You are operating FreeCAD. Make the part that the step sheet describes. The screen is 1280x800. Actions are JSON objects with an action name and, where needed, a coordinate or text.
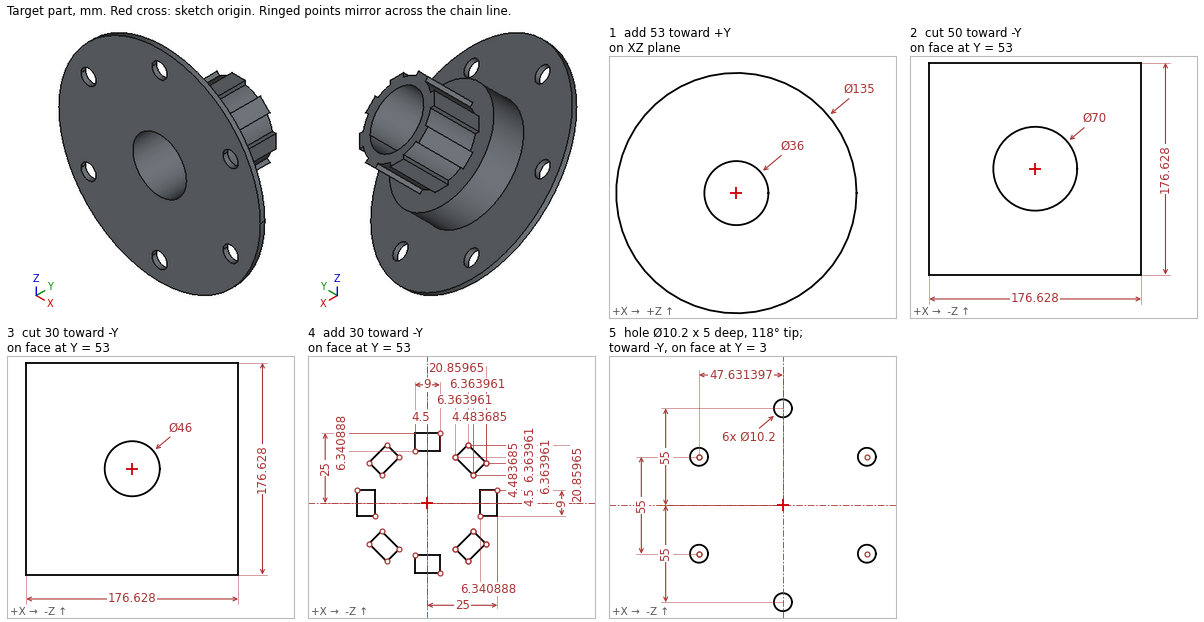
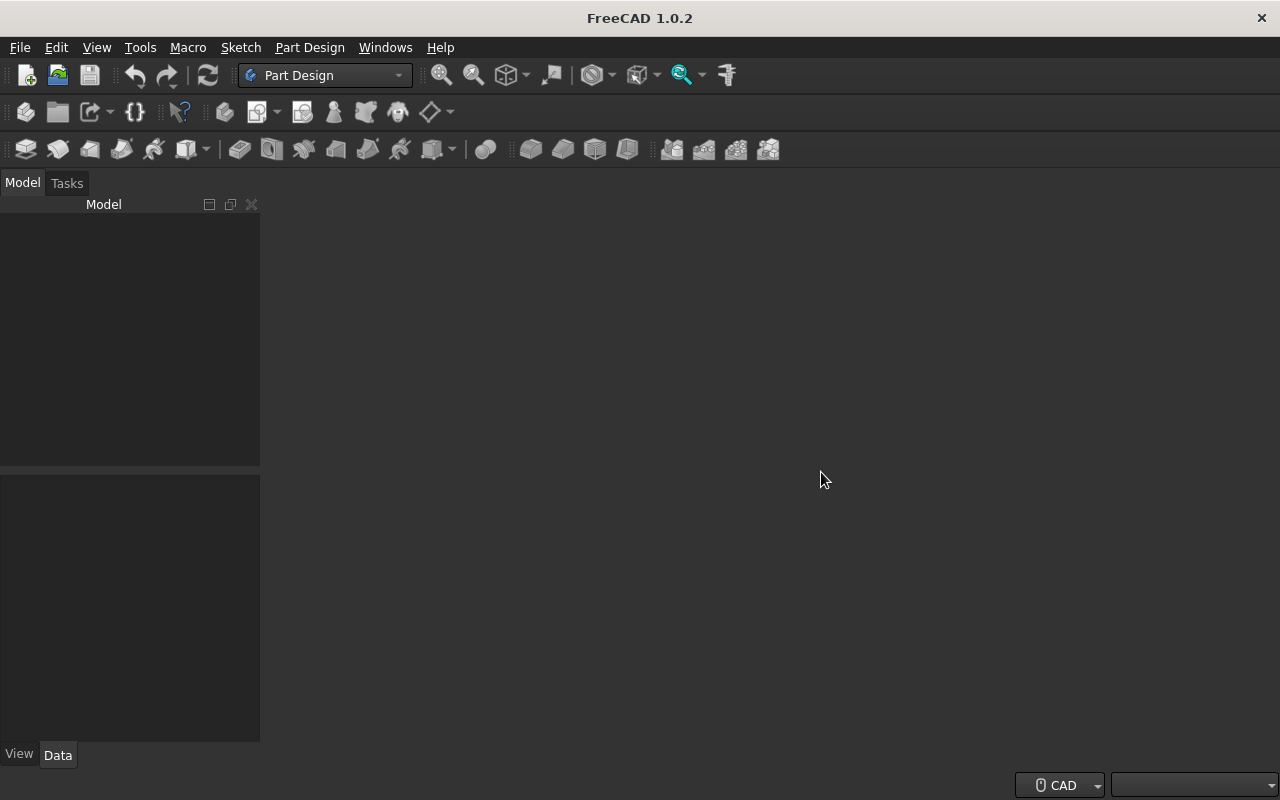
{"action": "left_click", "coordinate": [26, 76]}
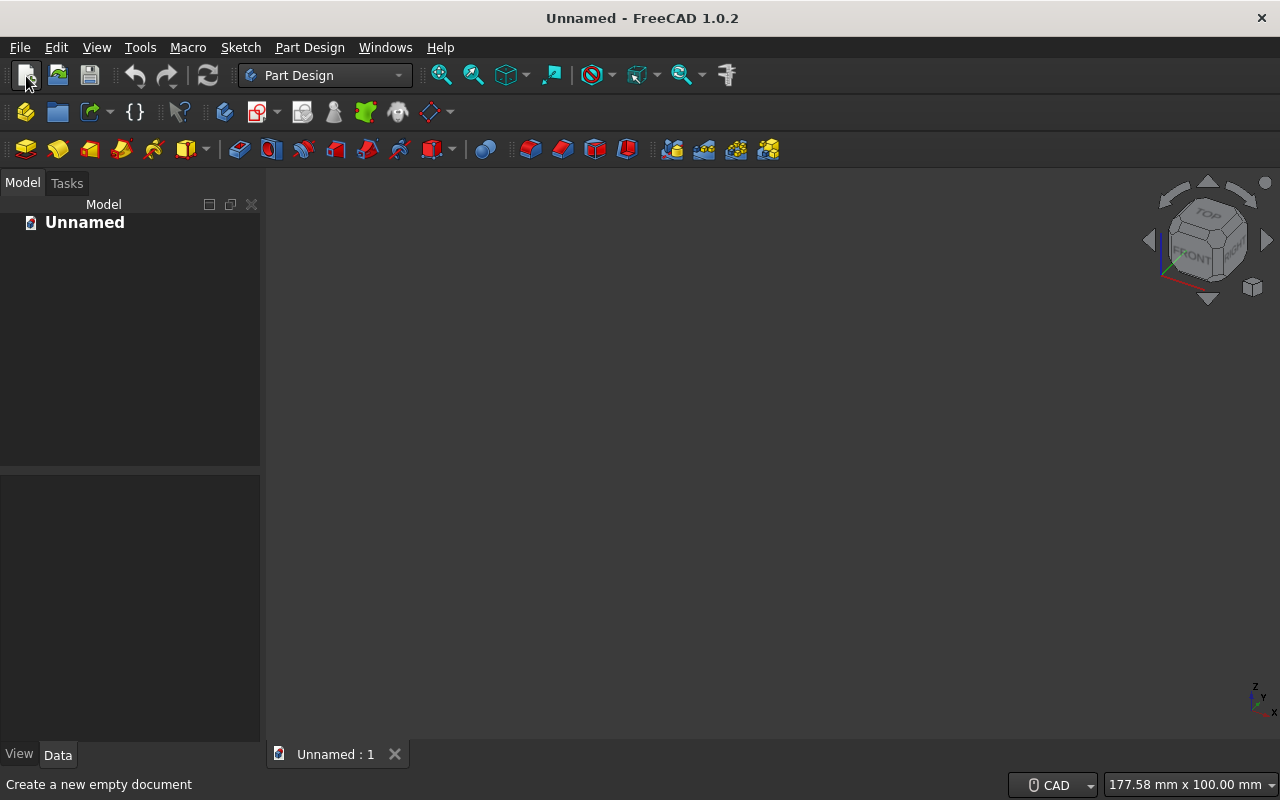
{"action": "left_click", "coordinate": [258, 112]}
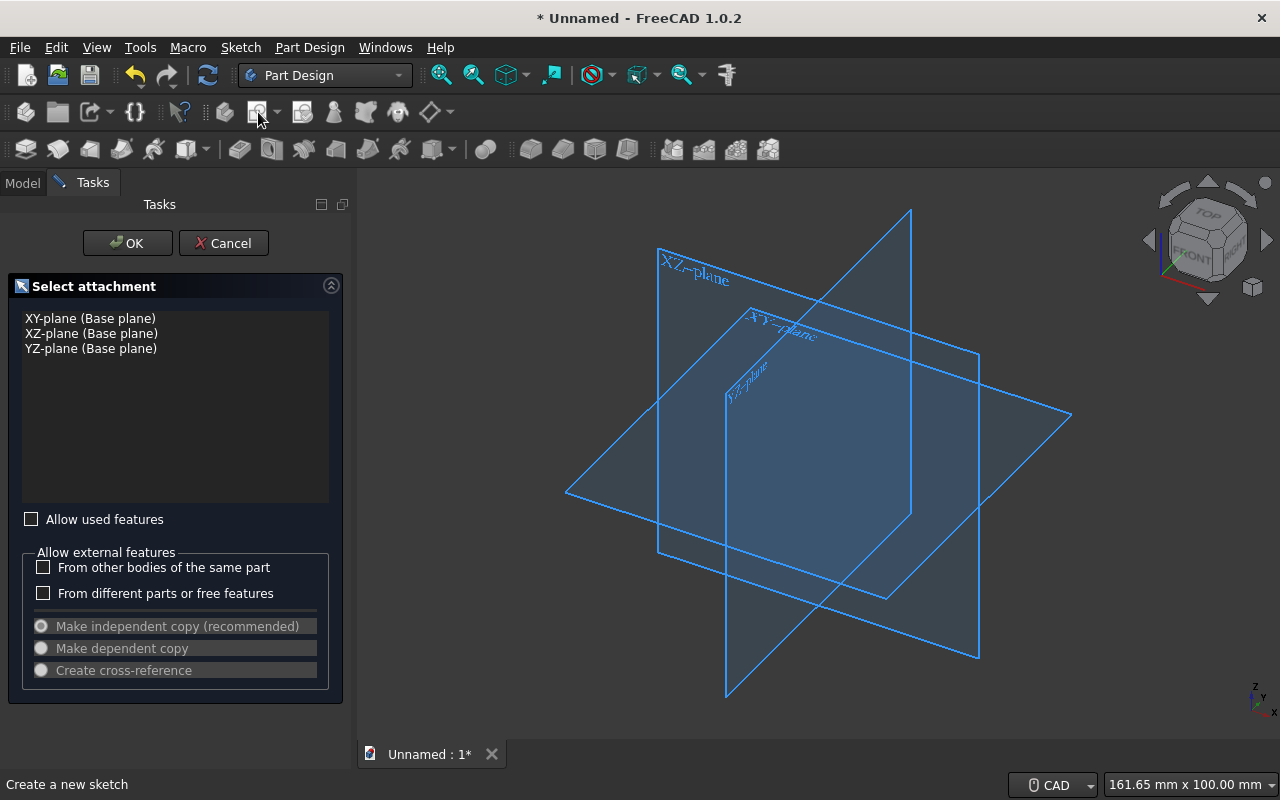
{"action": "left_click", "coordinate": [82, 334]}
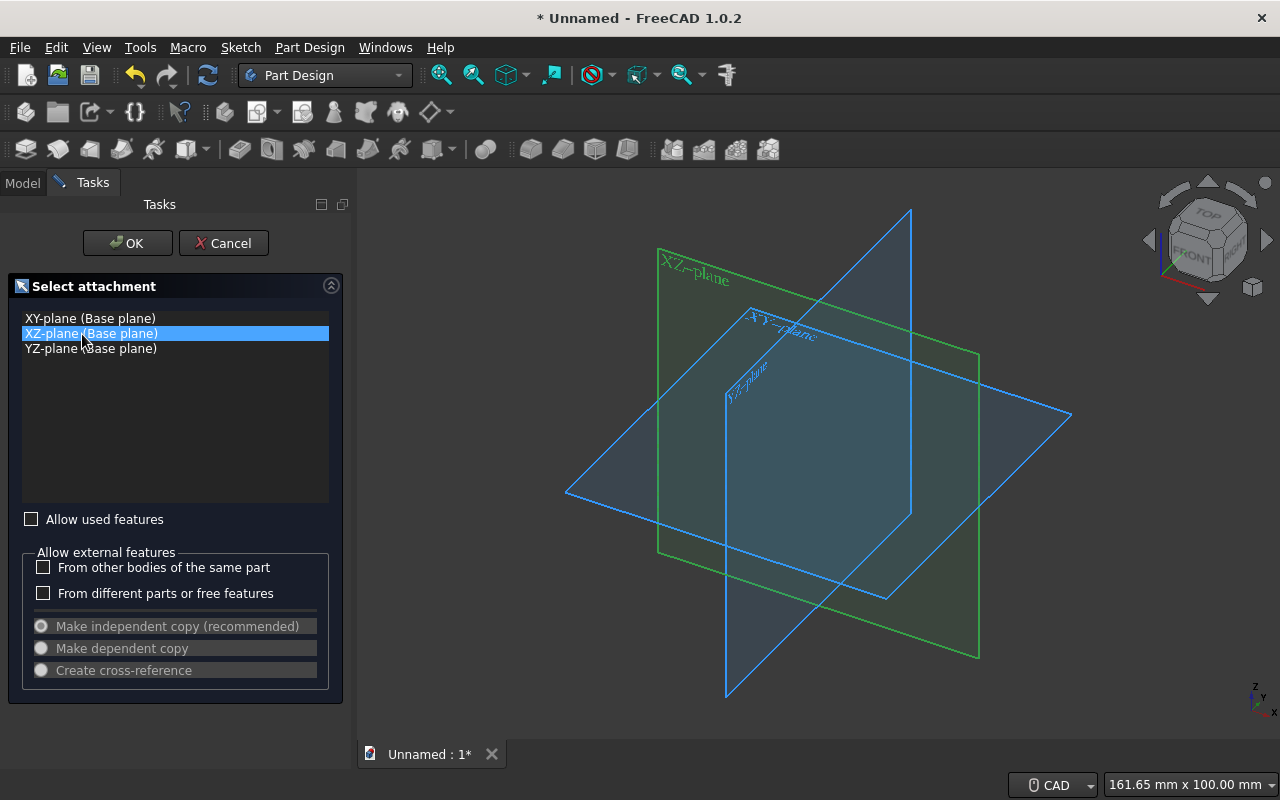
{"action": "left_click", "coordinate": [128, 243]}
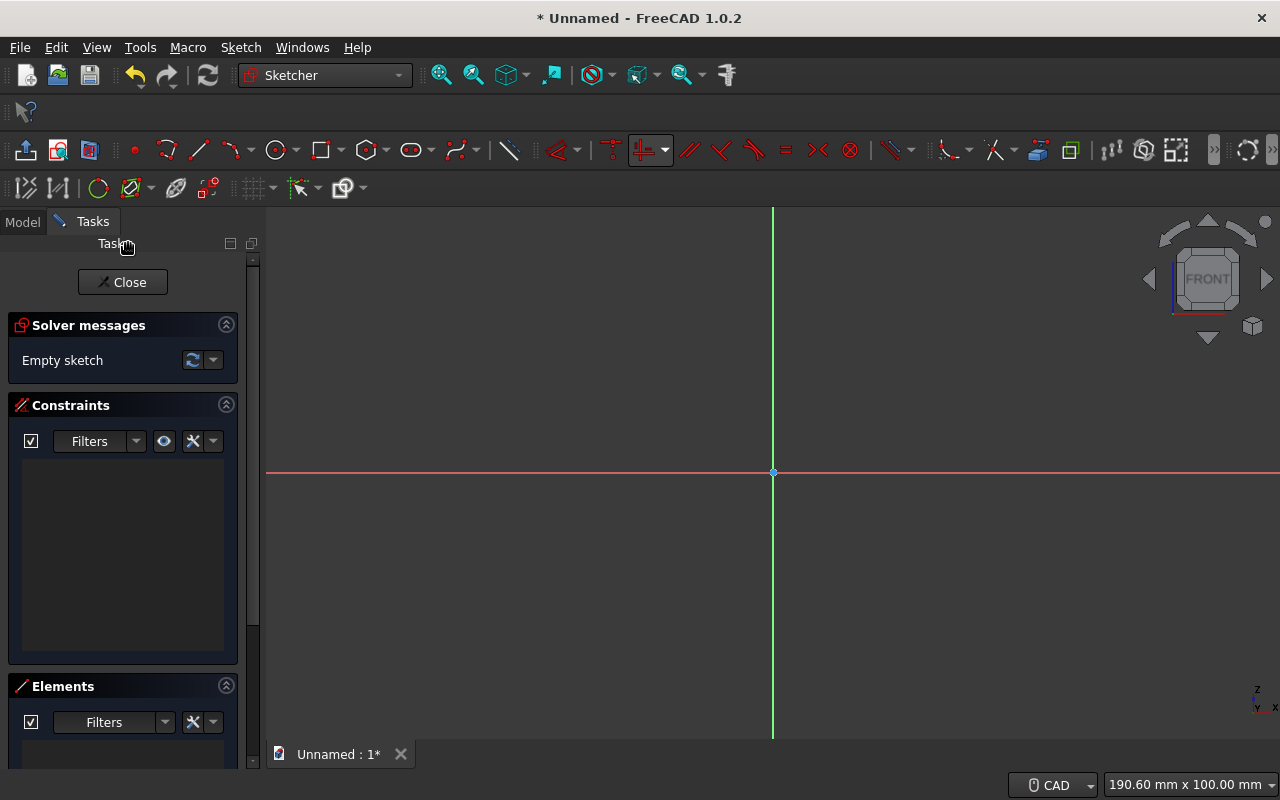
{"action": "scroll", "coordinate": [649, 473], "scroll_direction": "down", "scroll_amount": 4}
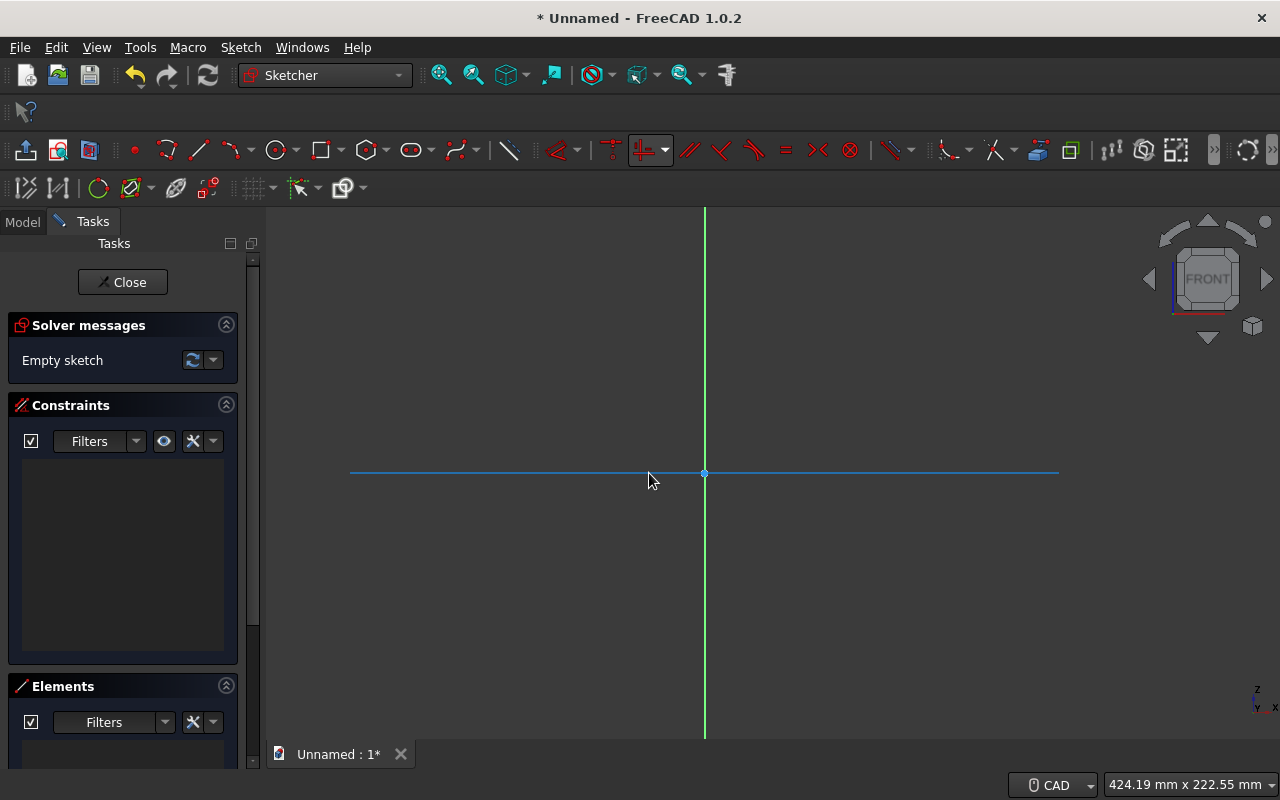
{"action": "left_click", "coordinate": [276, 150]}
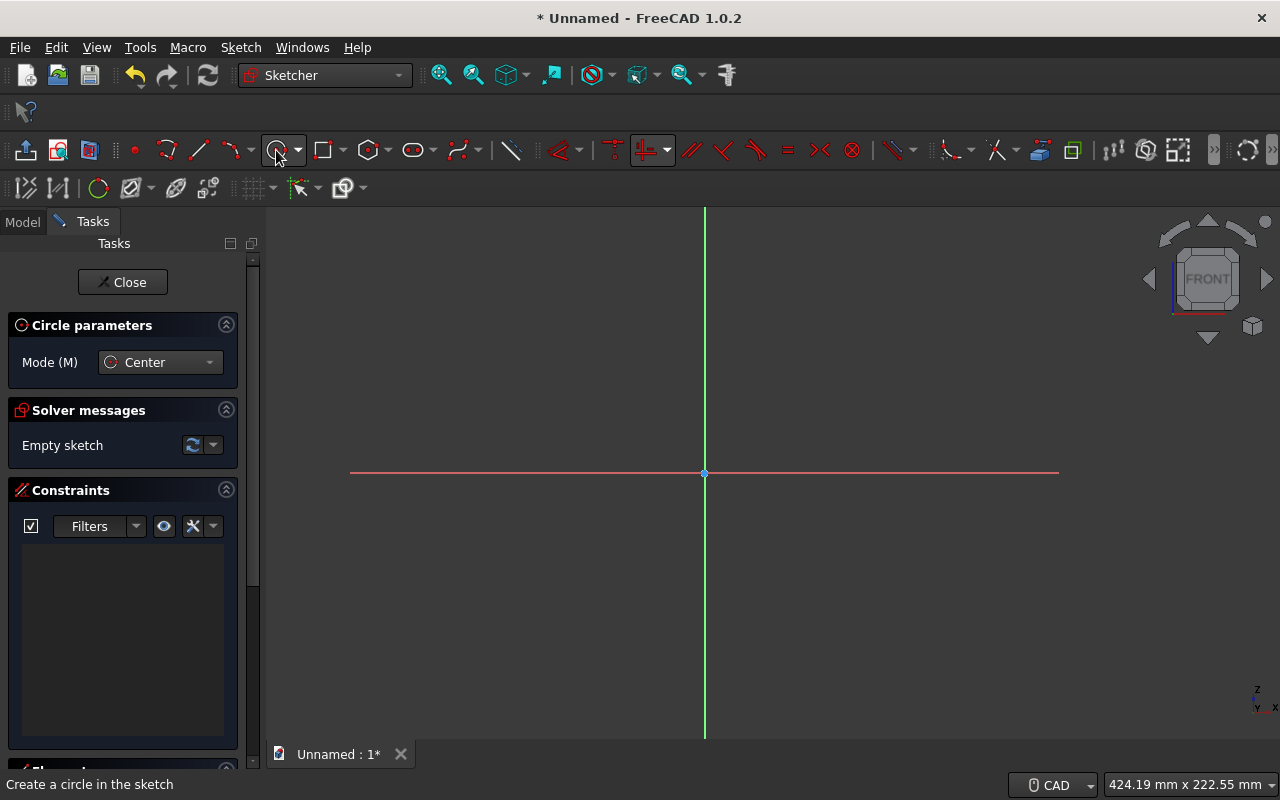
{"action": "left_click", "coordinate": [705, 473]}
{"action": "left_click", "coordinate": [819, 359]}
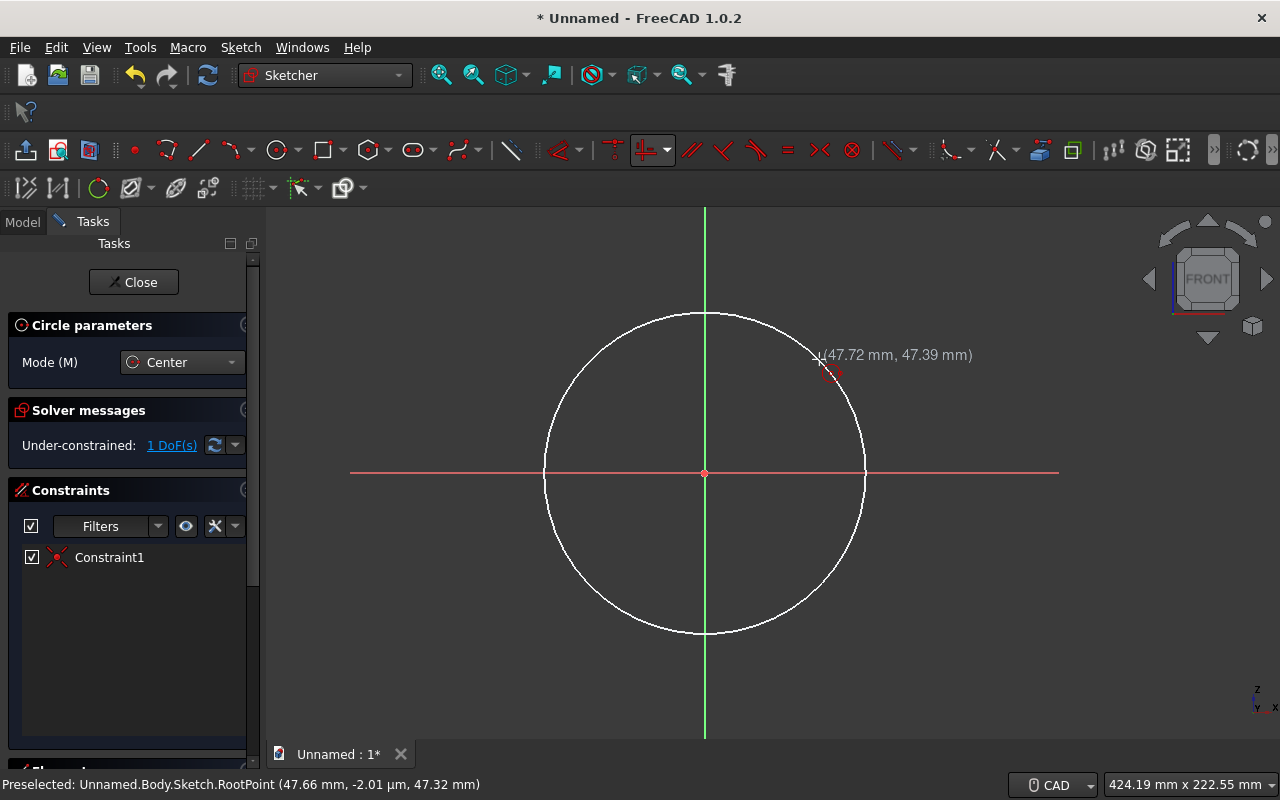
{"action": "left_click", "coordinate": [705, 473]}
{"action": "left_click", "coordinate": [735, 443]}
{"action": "key", "text": "Escape"}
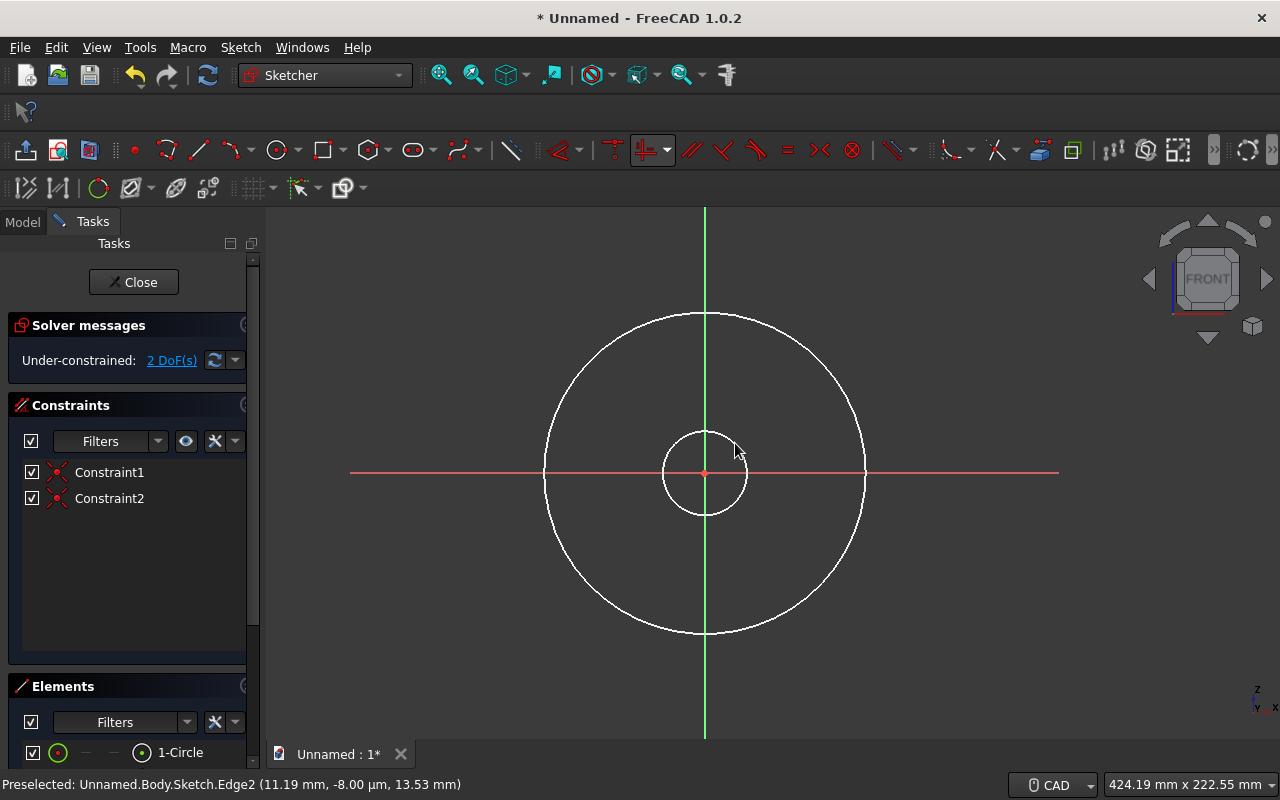
{"action": "left_click", "coordinate": [558, 150]}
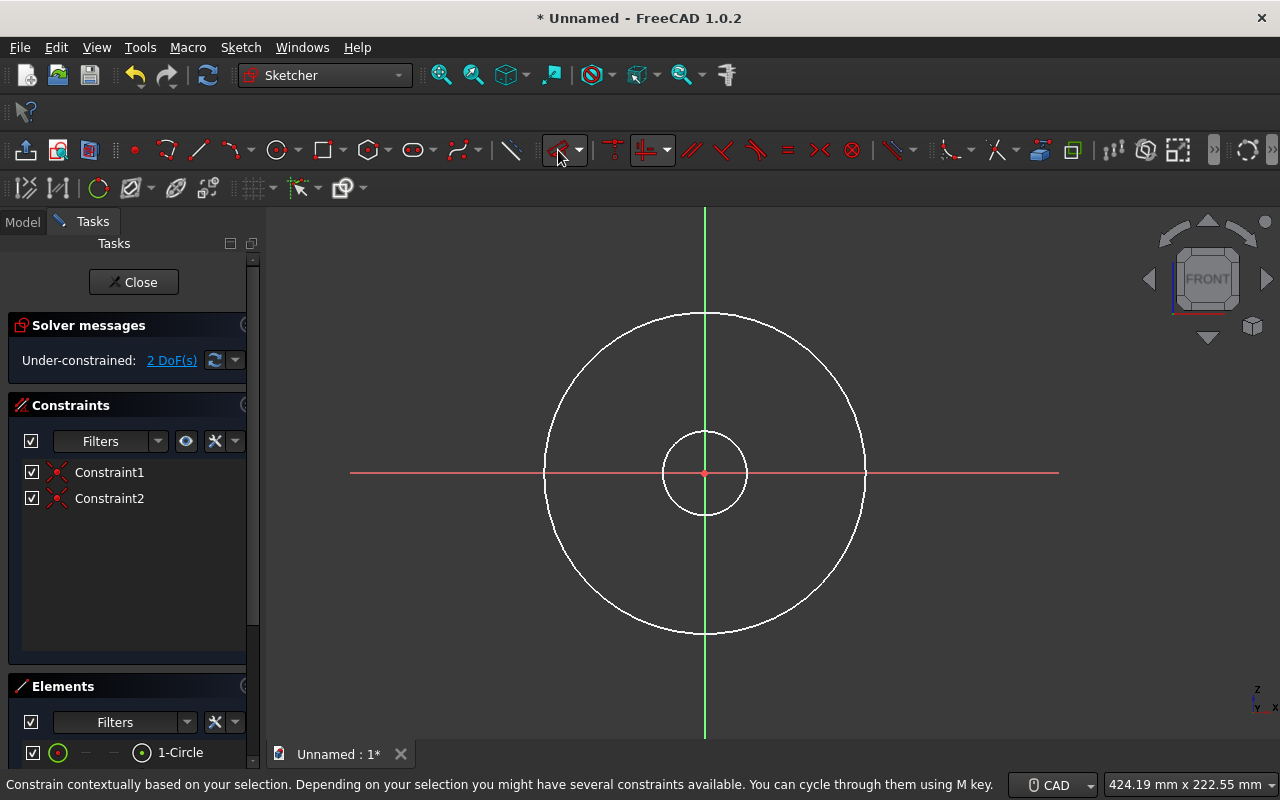
{"action": "left_click", "coordinate": [818, 359]}
{"action": "left_click", "coordinate": [841, 336]}